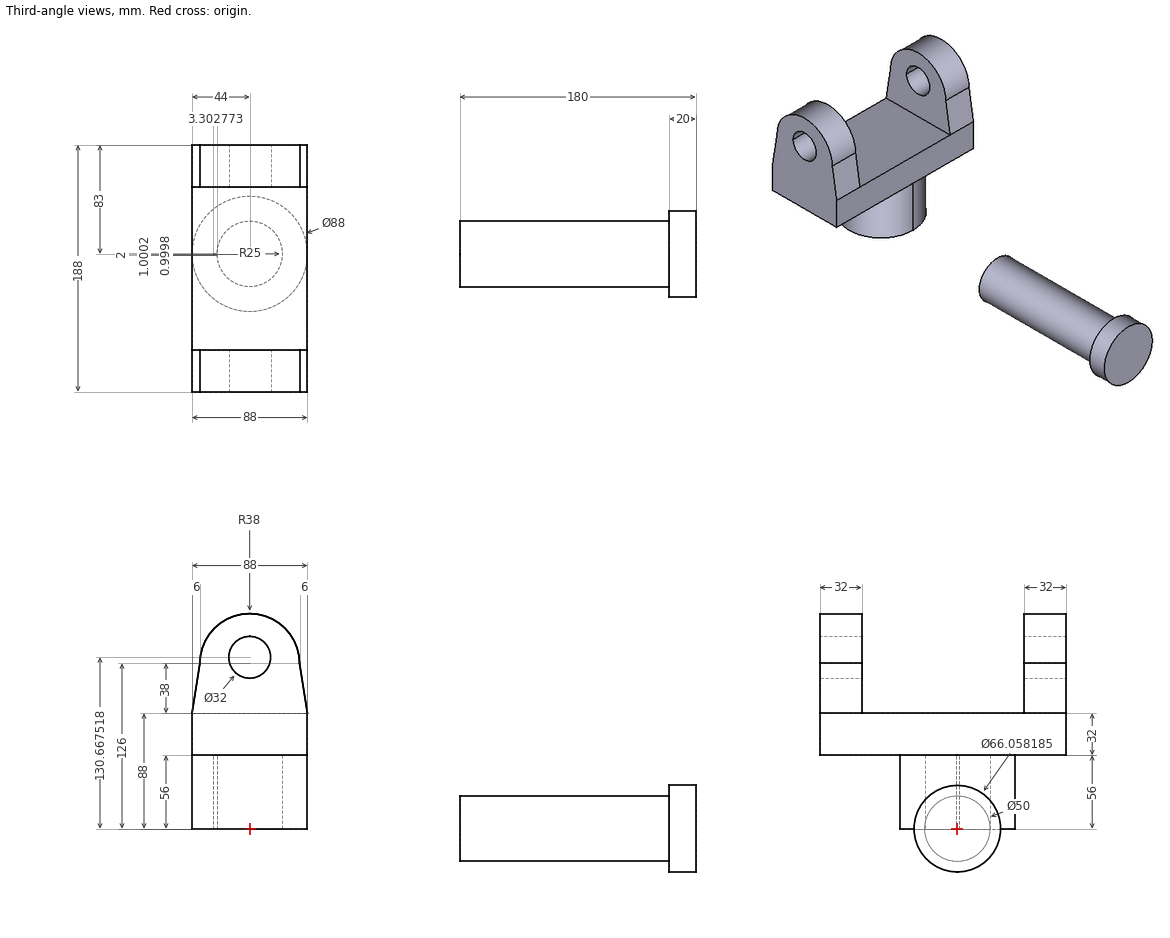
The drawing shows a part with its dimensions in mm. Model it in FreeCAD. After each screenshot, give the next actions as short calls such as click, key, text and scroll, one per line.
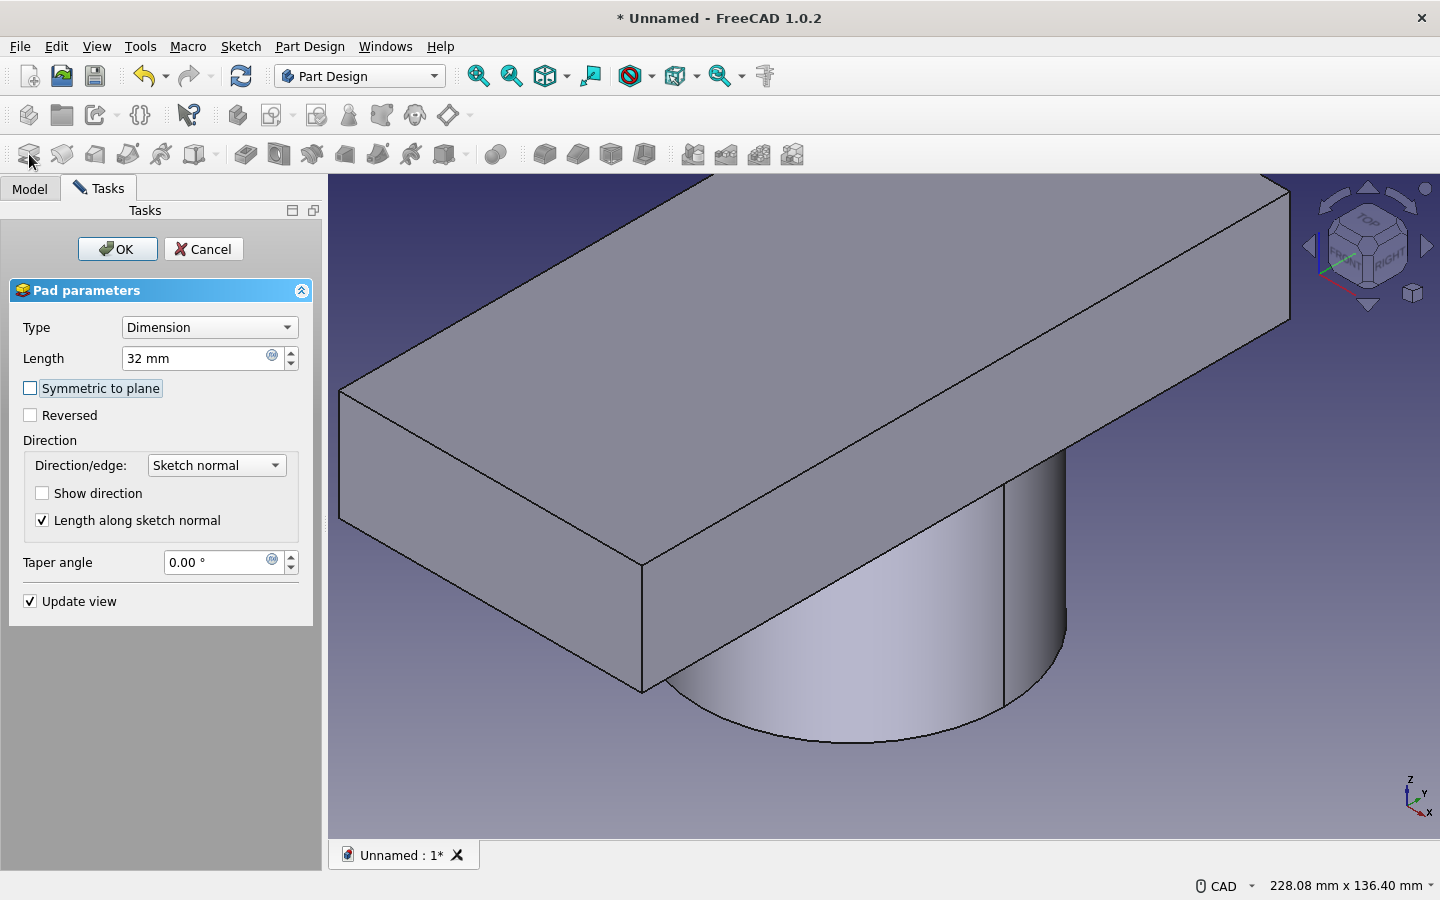
click(118, 249)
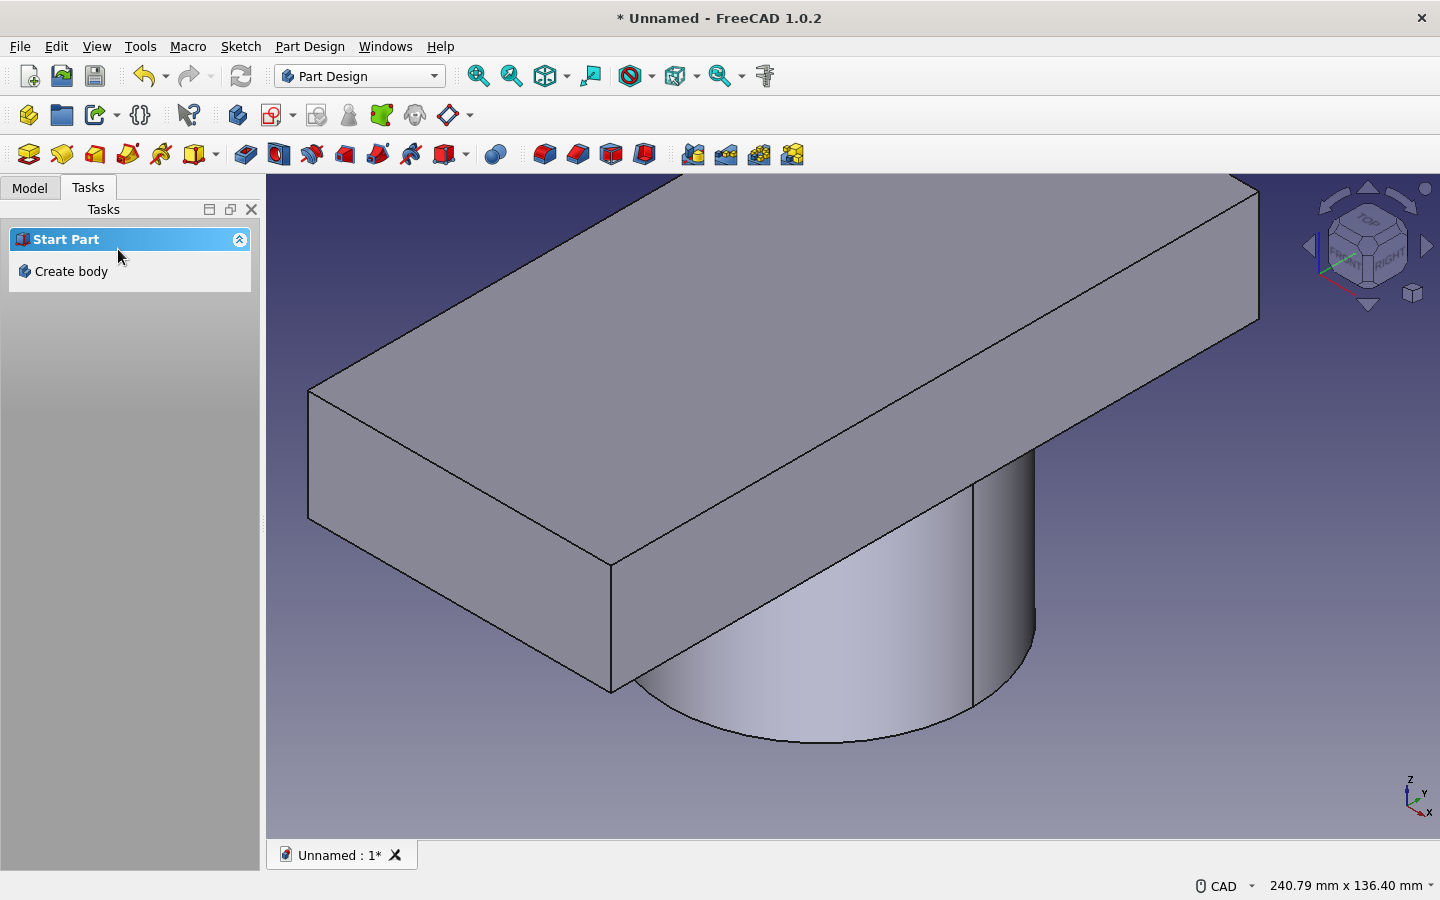
key(v)
key(f)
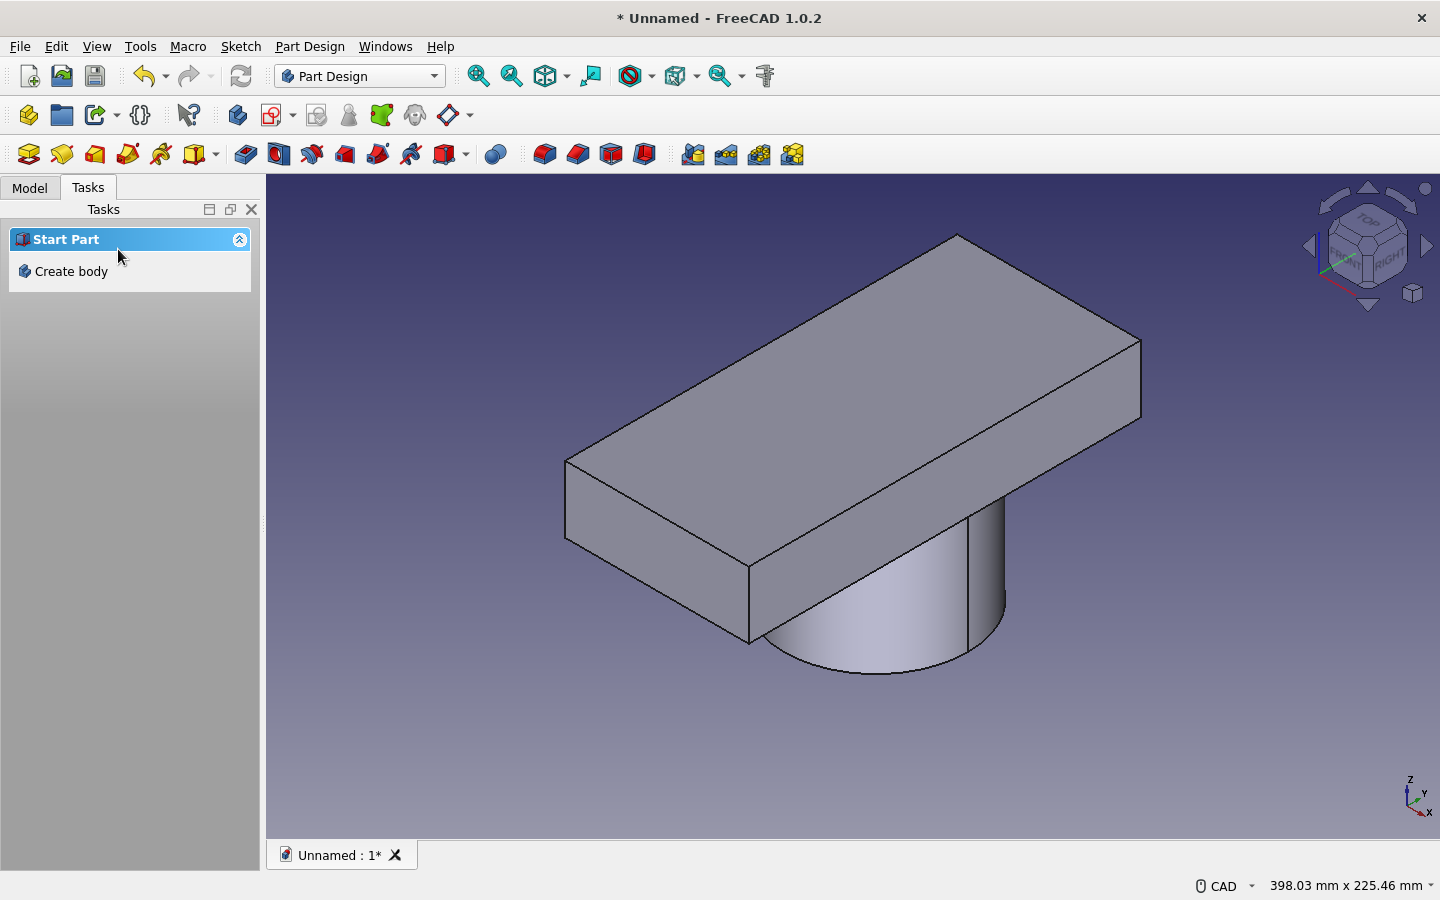
key(4)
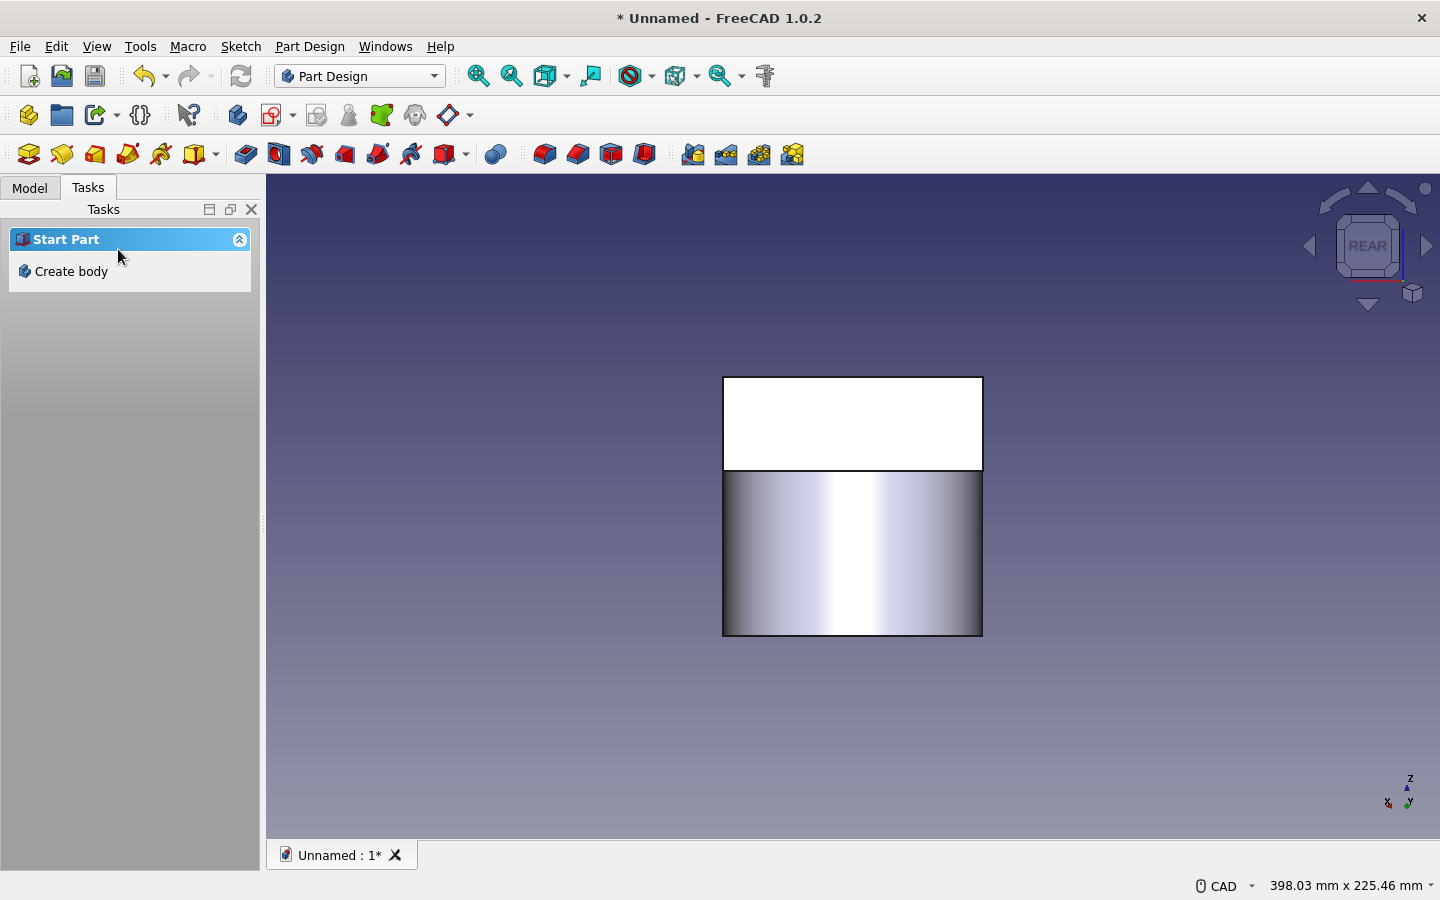
key(v)
key(f)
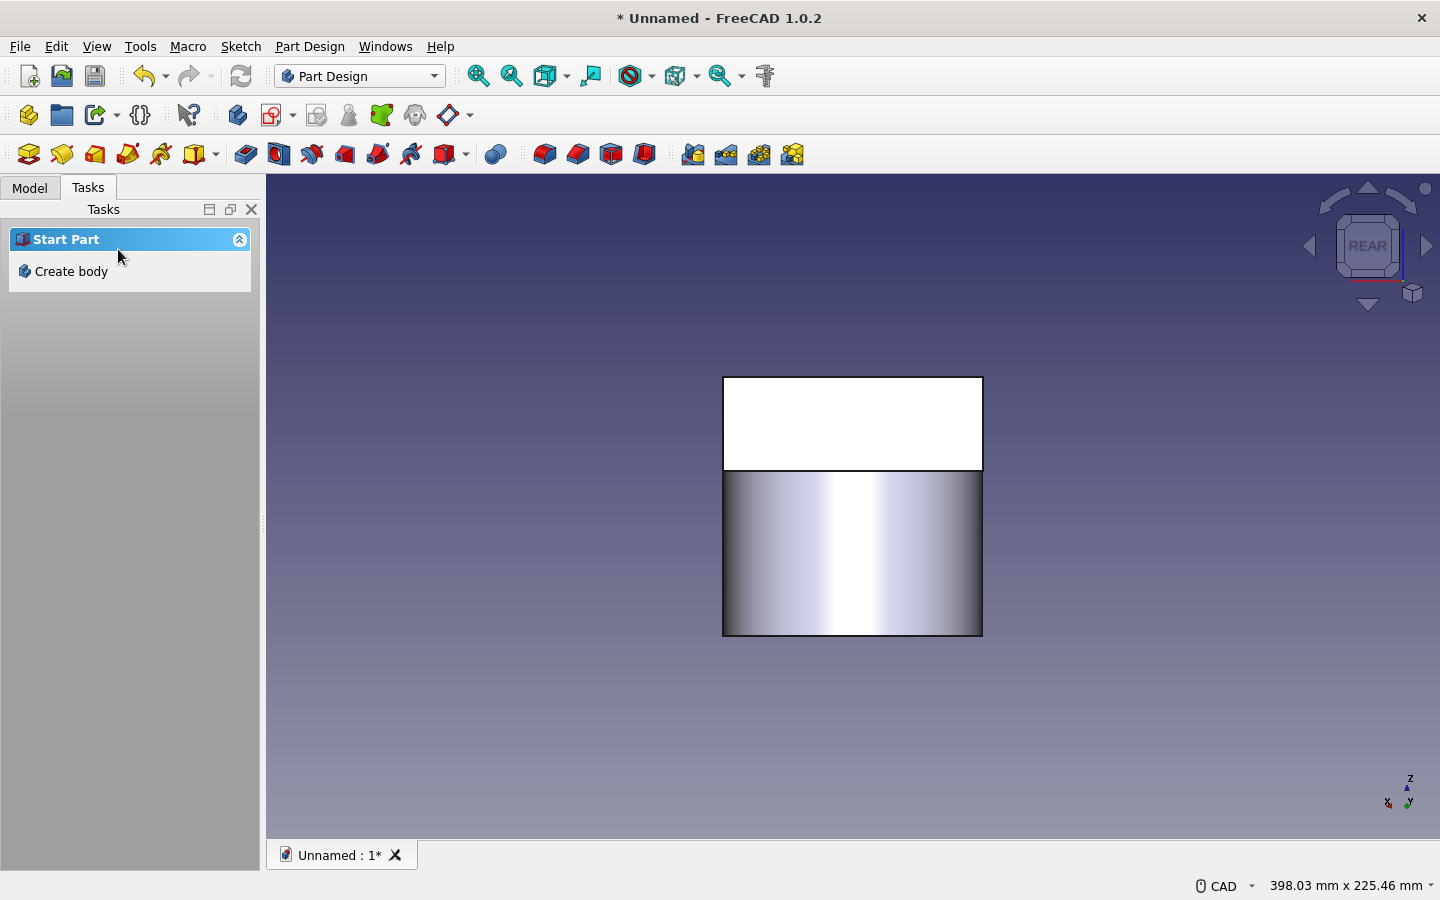
click(779, 423)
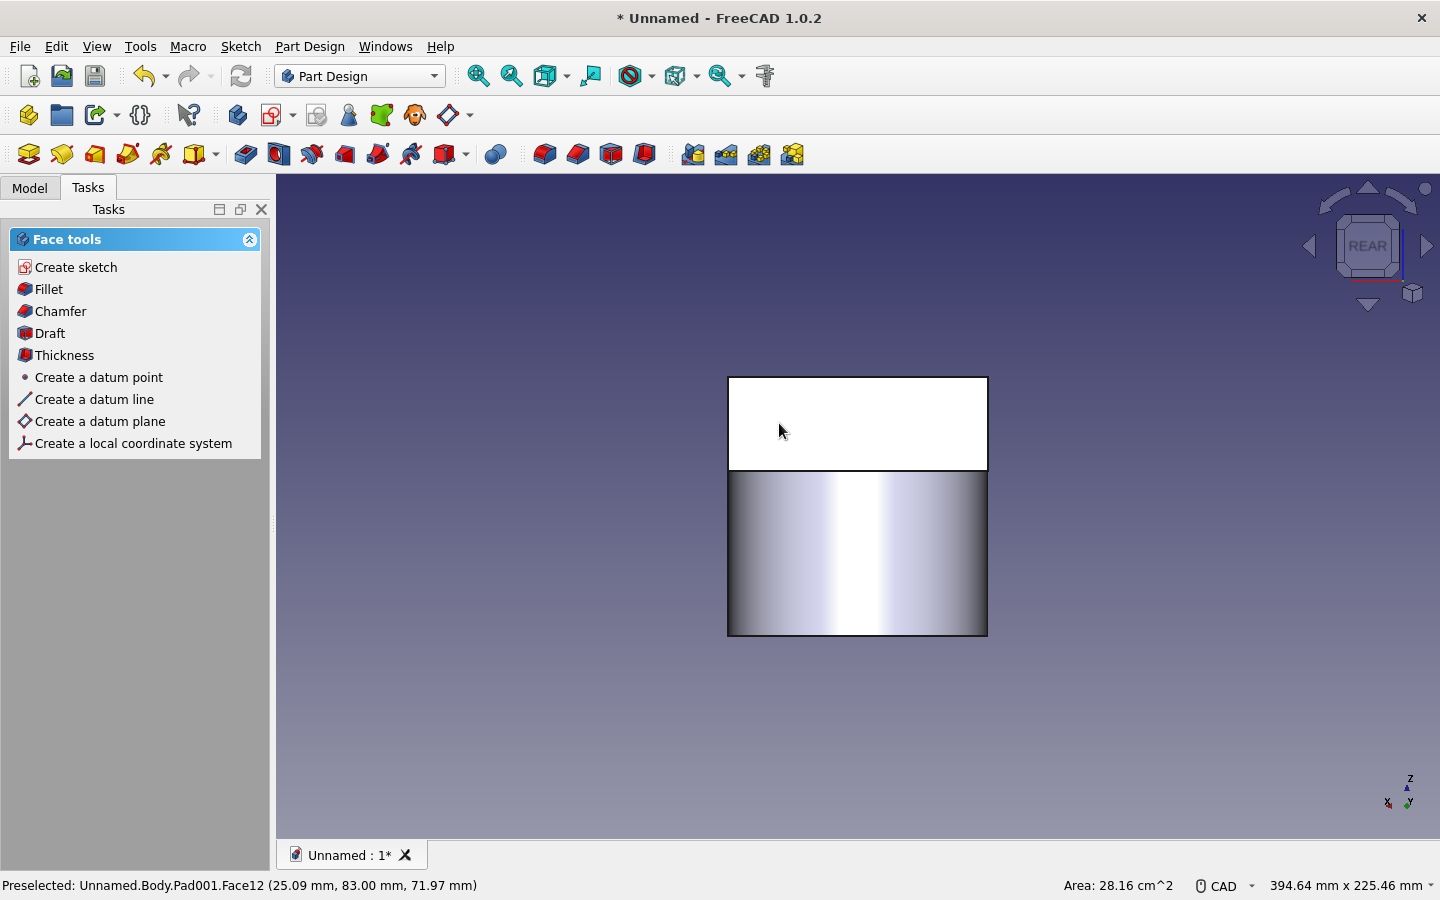
click(270, 116)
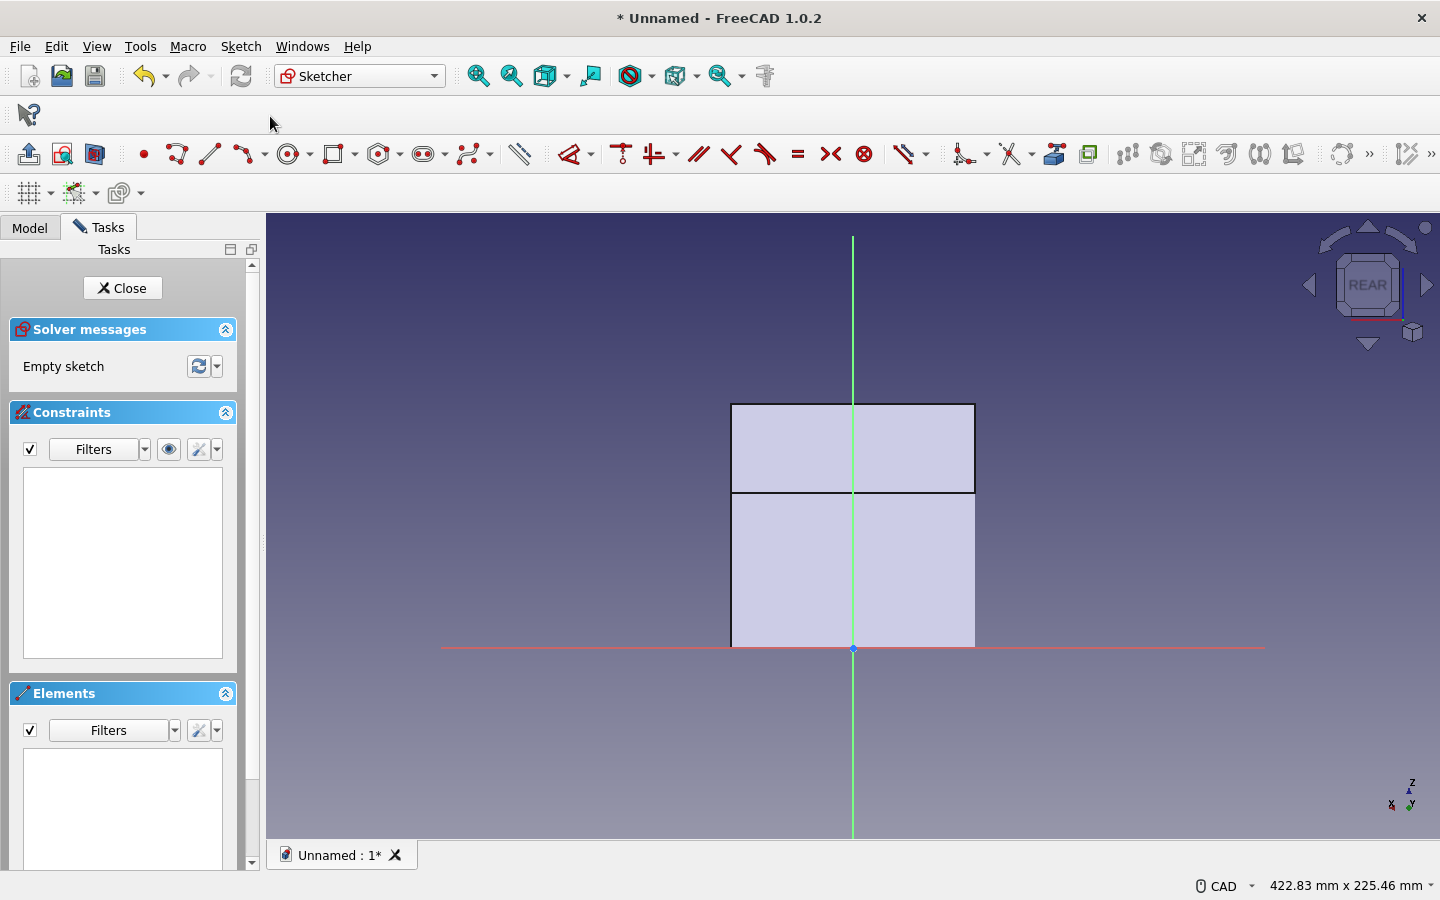
scroll(475, 811, down, 1)